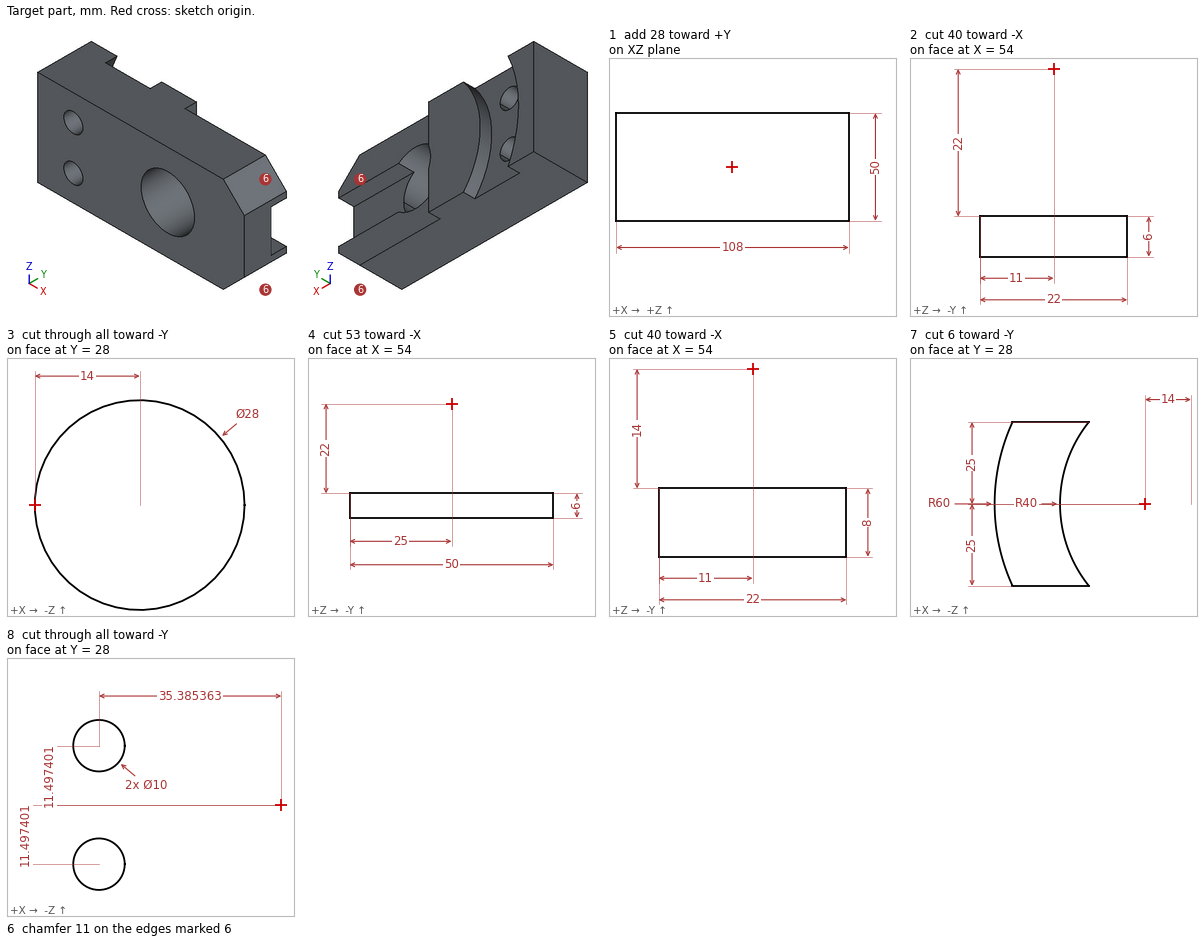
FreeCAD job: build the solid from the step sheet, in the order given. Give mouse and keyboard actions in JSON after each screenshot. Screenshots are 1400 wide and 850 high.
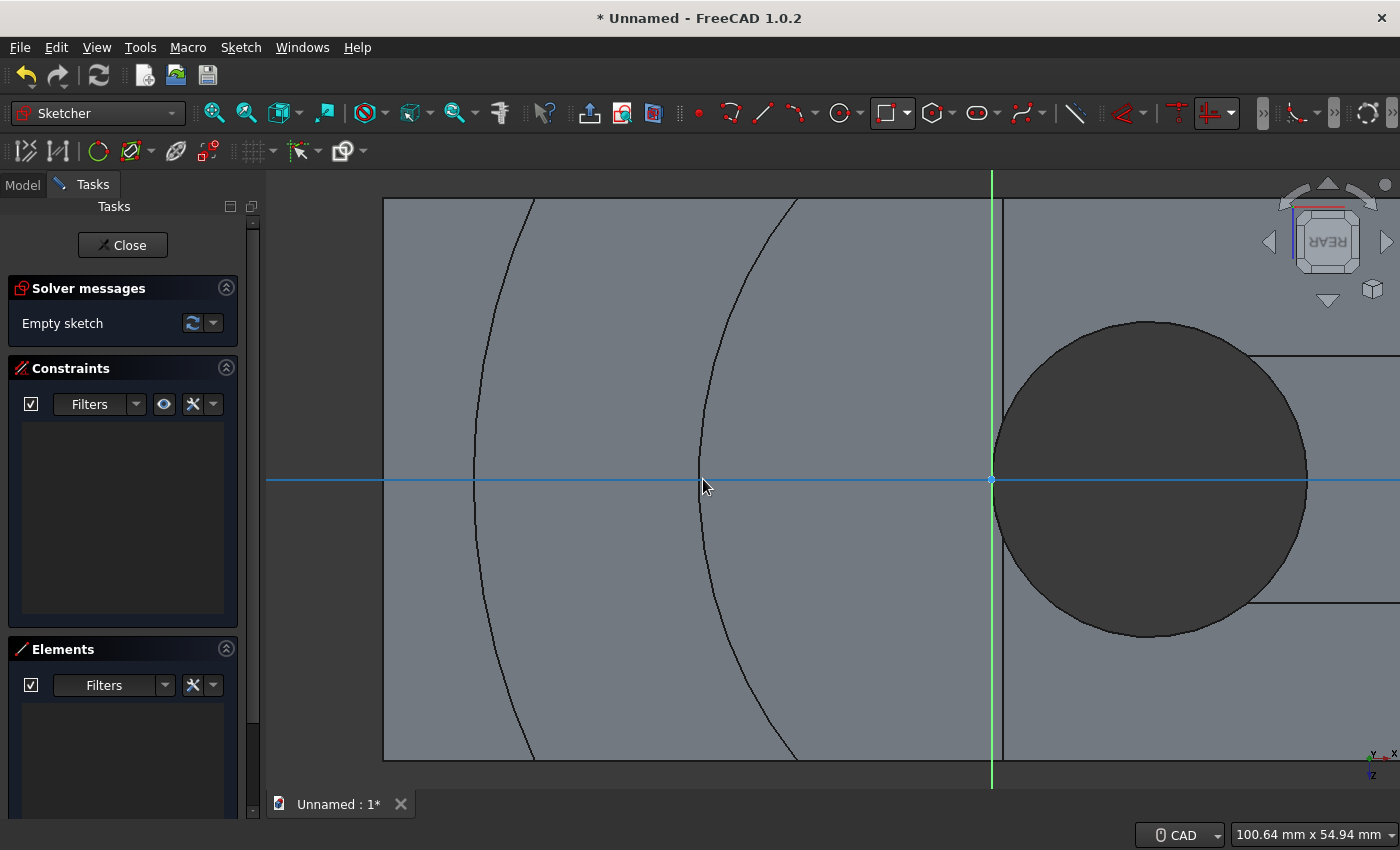
{"action": "key", "text": "g c"}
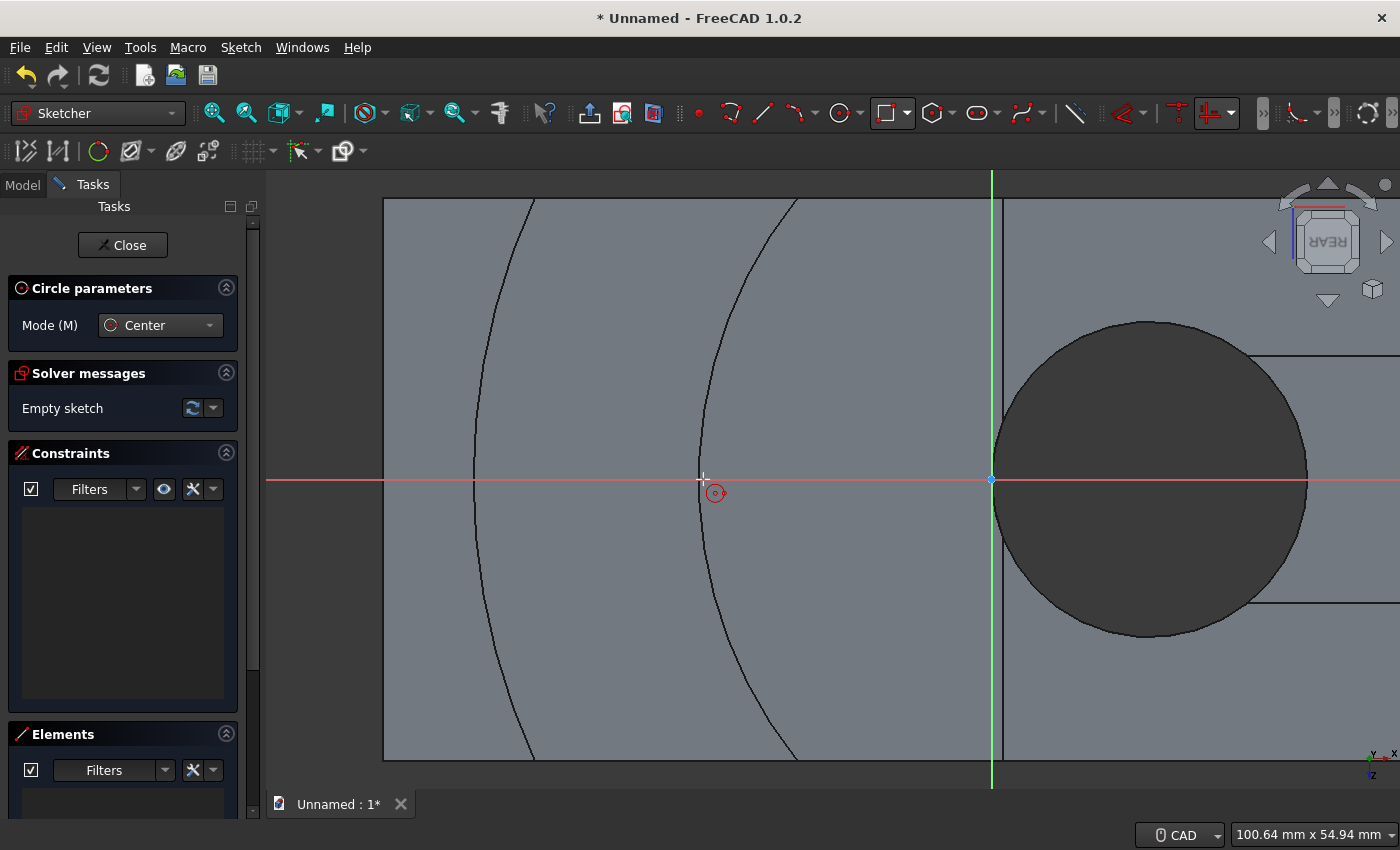
{"action": "left_click", "coordinate": [593, 350]}
{"action": "mouse_move", "coordinate": [633, 310]}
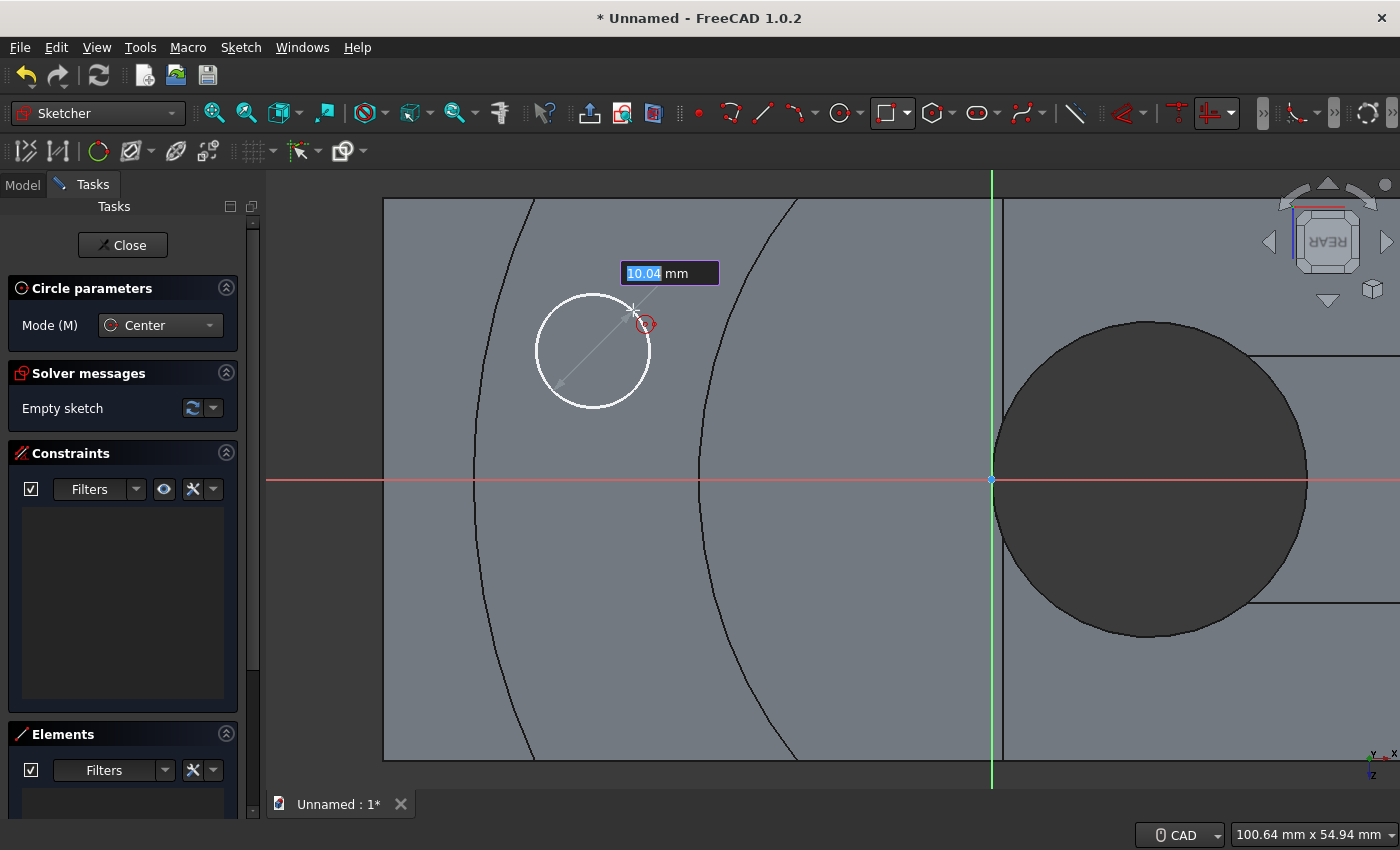
{"action": "type", "text": "10"}
{"action": "key", "text": "Return"}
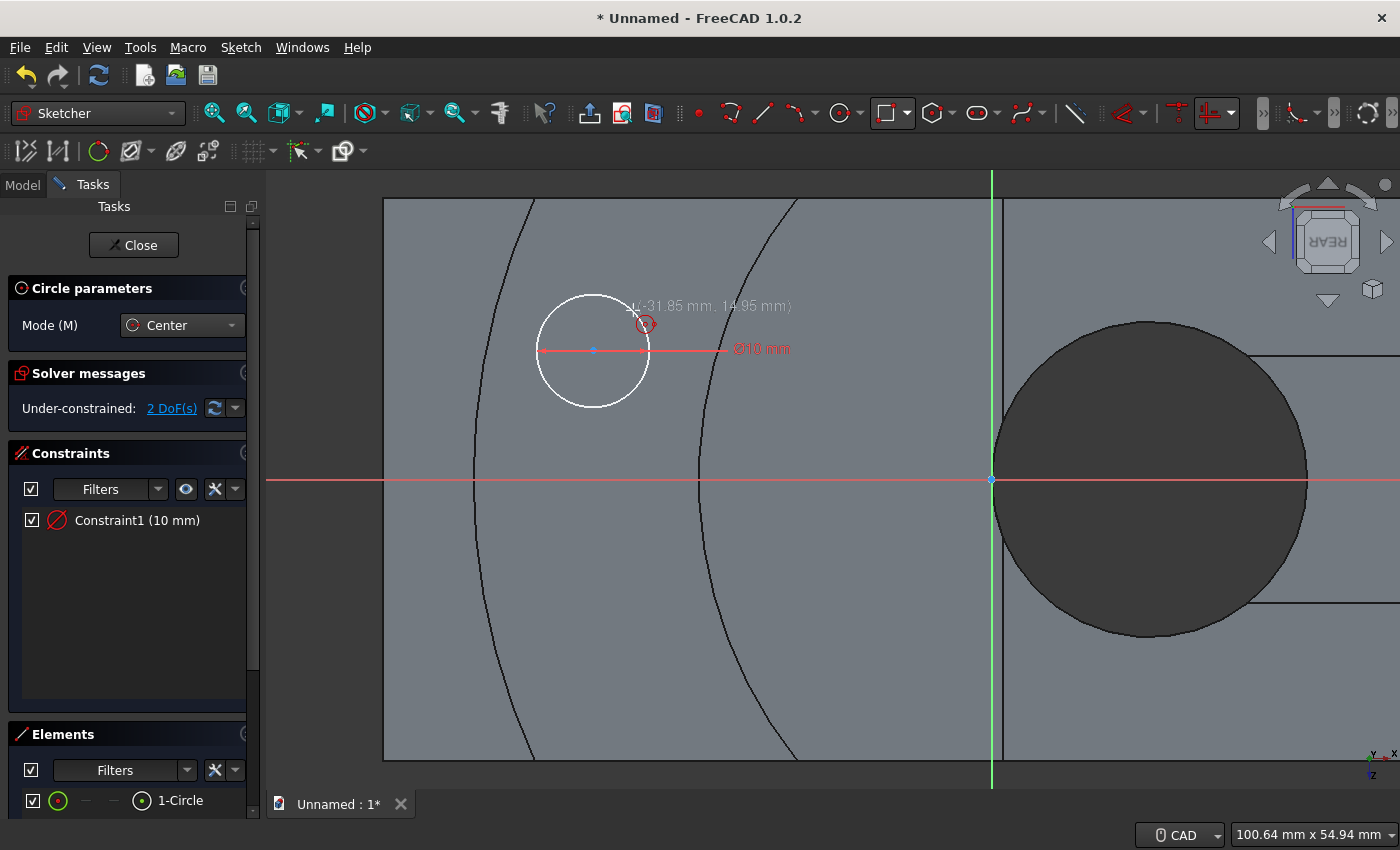
{"action": "left_click", "coordinate": [593, 609]}
{"action": "mouse_move", "coordinate": [633, 569]}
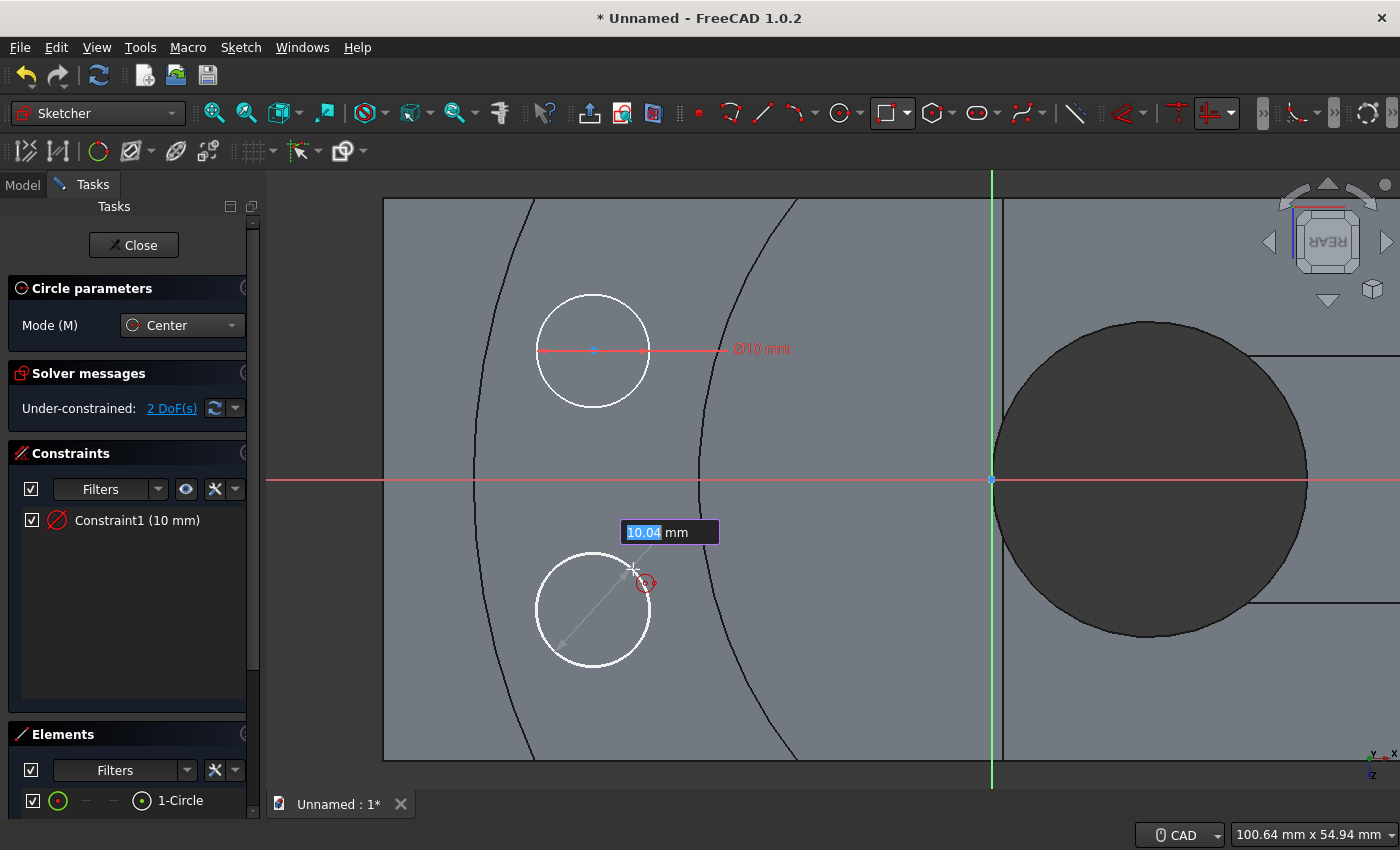
{"action": "type", "text": "10"}
{"action": "key", "text": "Return"}
{"action": "key", "text": "Escape"}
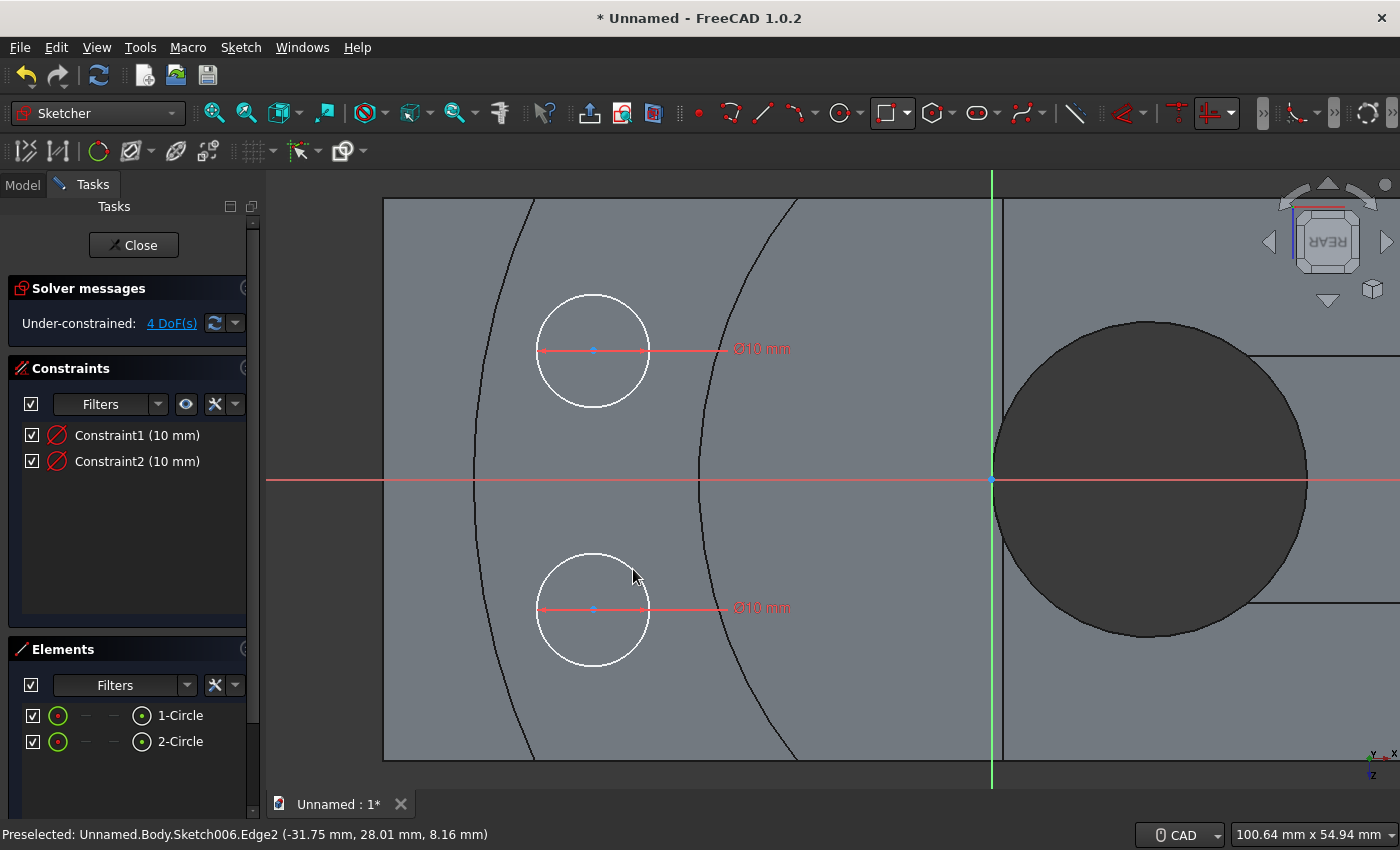
{"action": "left_click", "coordinate": [593, 351]}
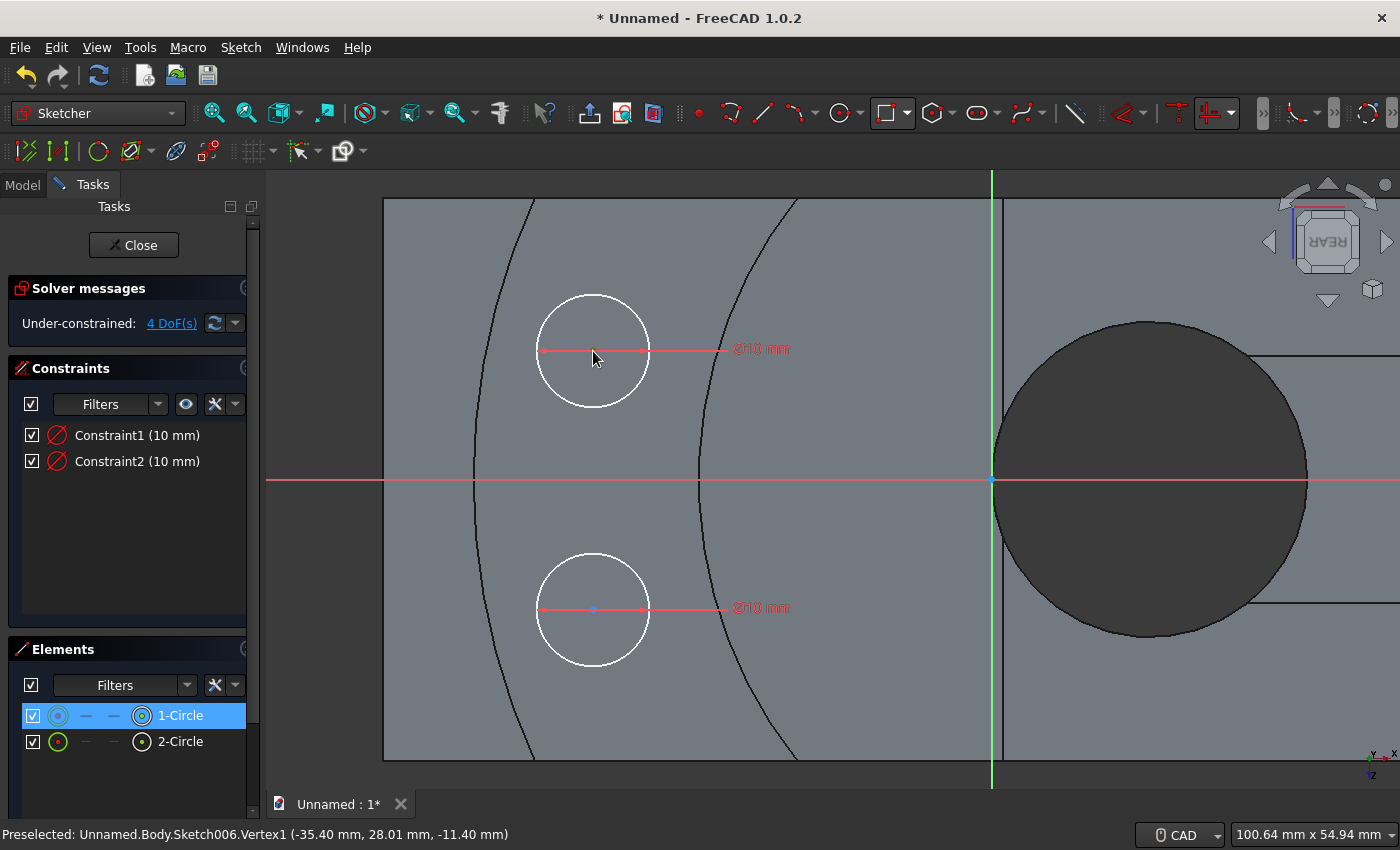
{"action": "left_click", "coordinate": [593, 610]}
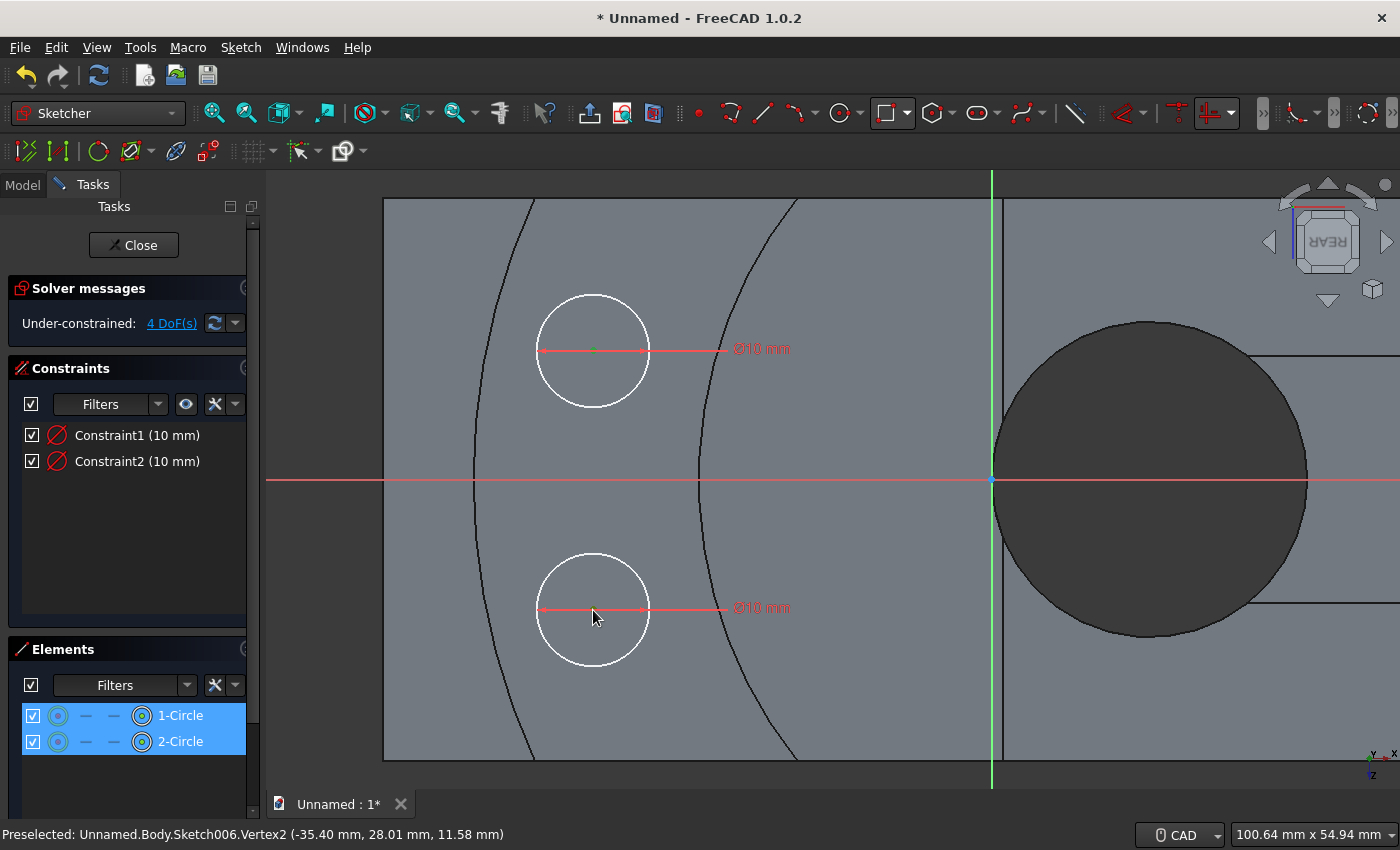
{"action": "key", "text": "v"}